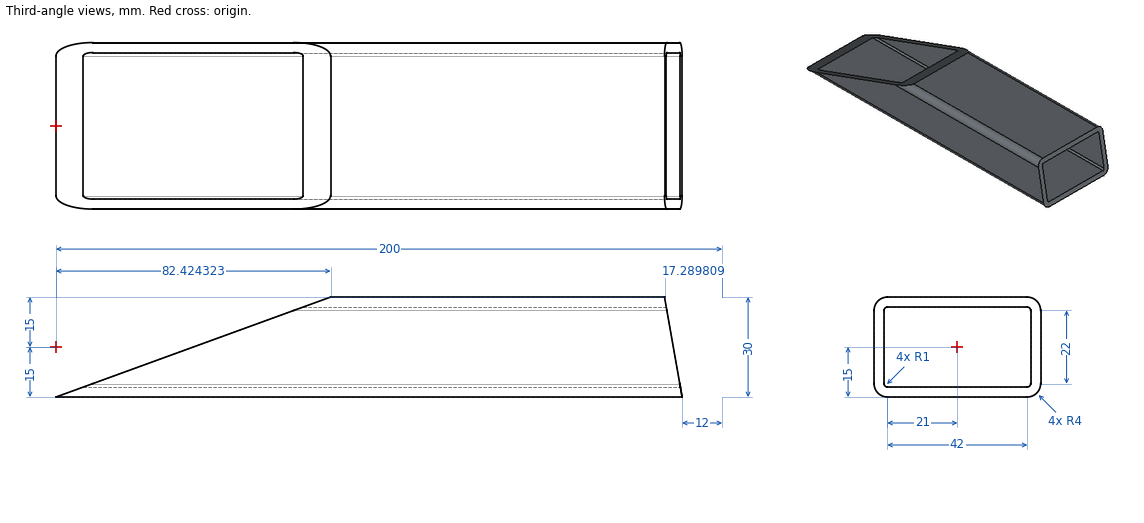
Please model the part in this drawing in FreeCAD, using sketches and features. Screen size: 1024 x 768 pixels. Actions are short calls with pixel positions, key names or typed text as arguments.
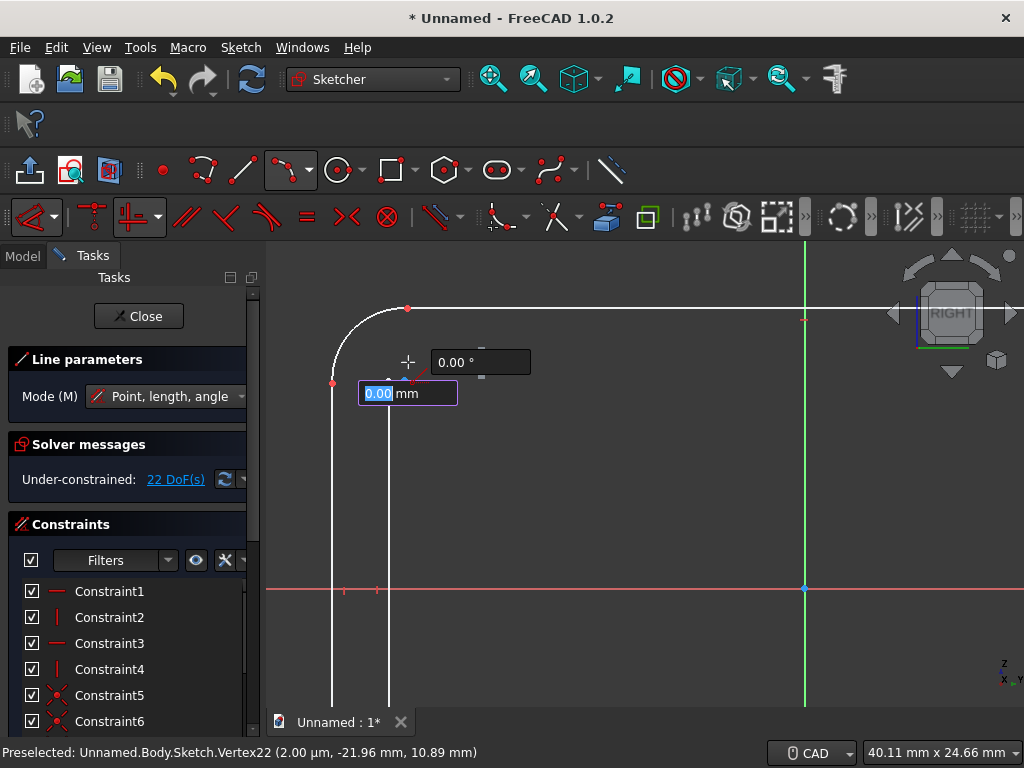
scroll(390, 380, down, 4)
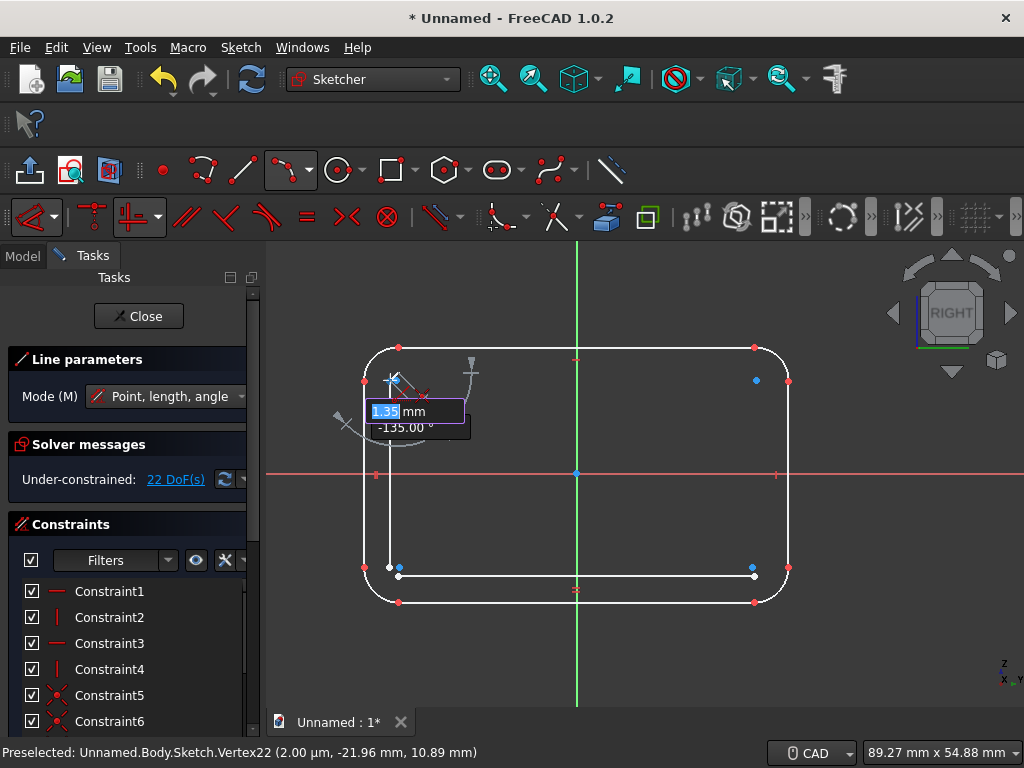
scroll(755, 372, up, 4)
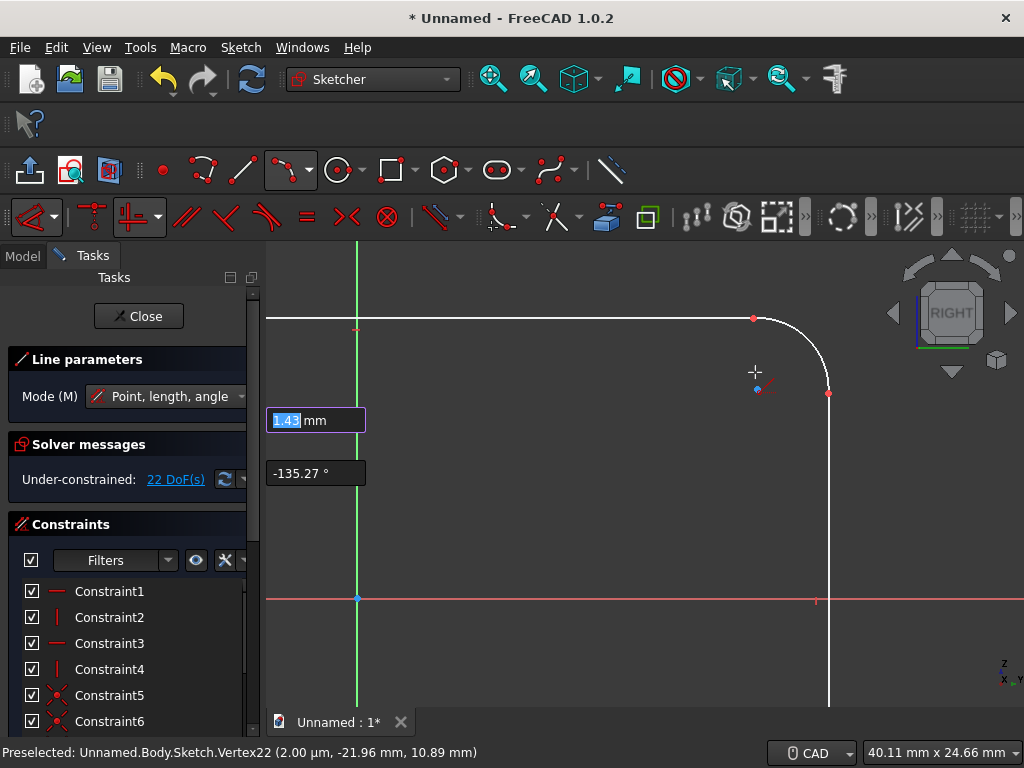
click(754, 372)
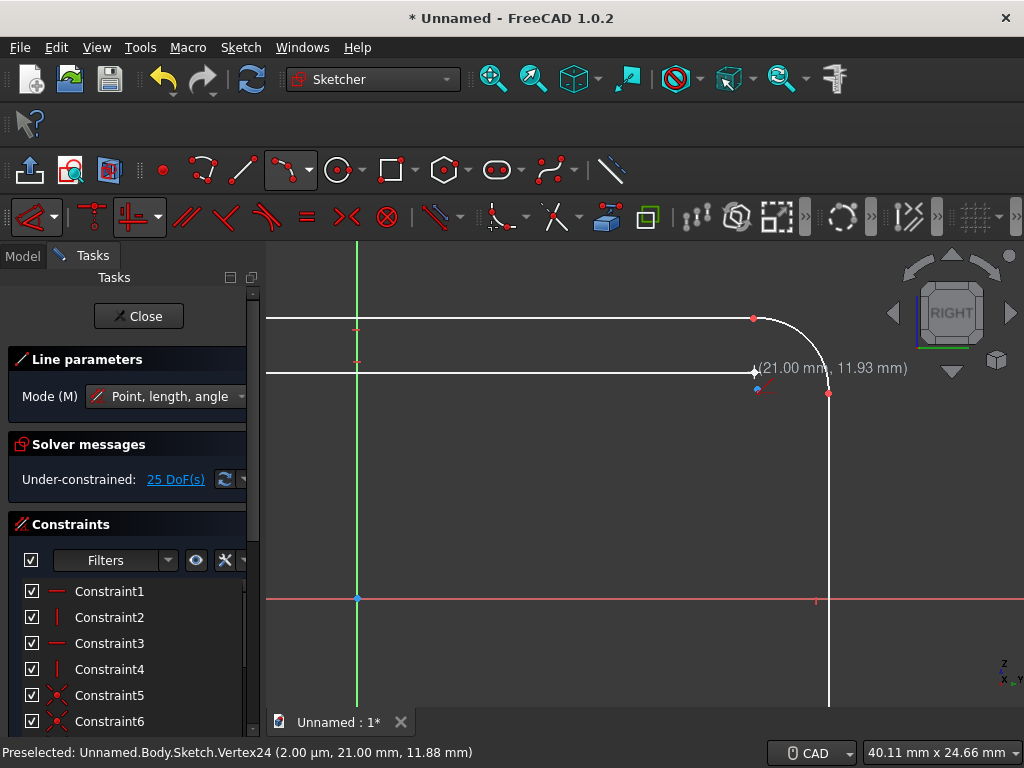
click(773, 391)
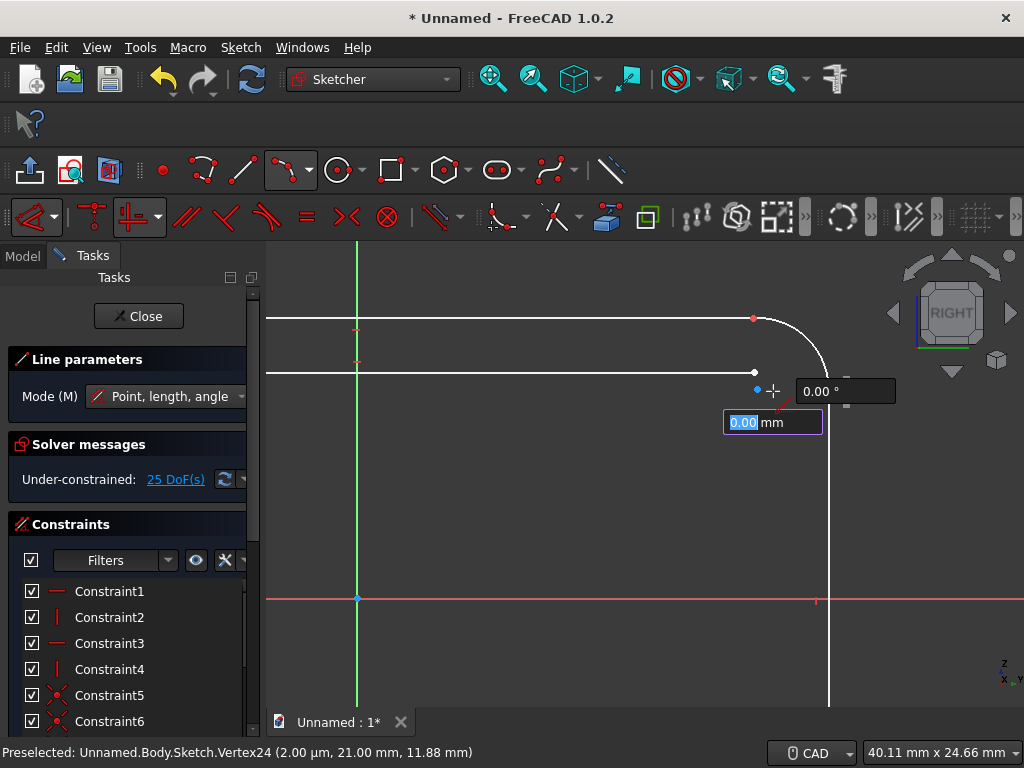
scroll(756, 372, down, 4)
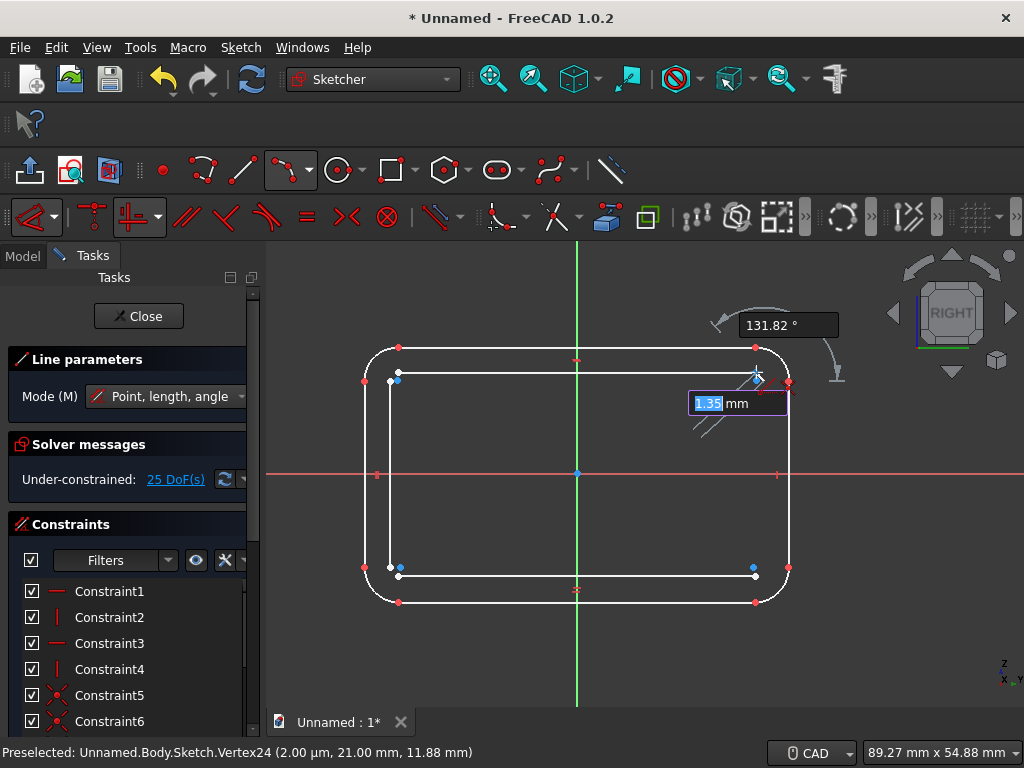
scroll(764, 567, up, 4)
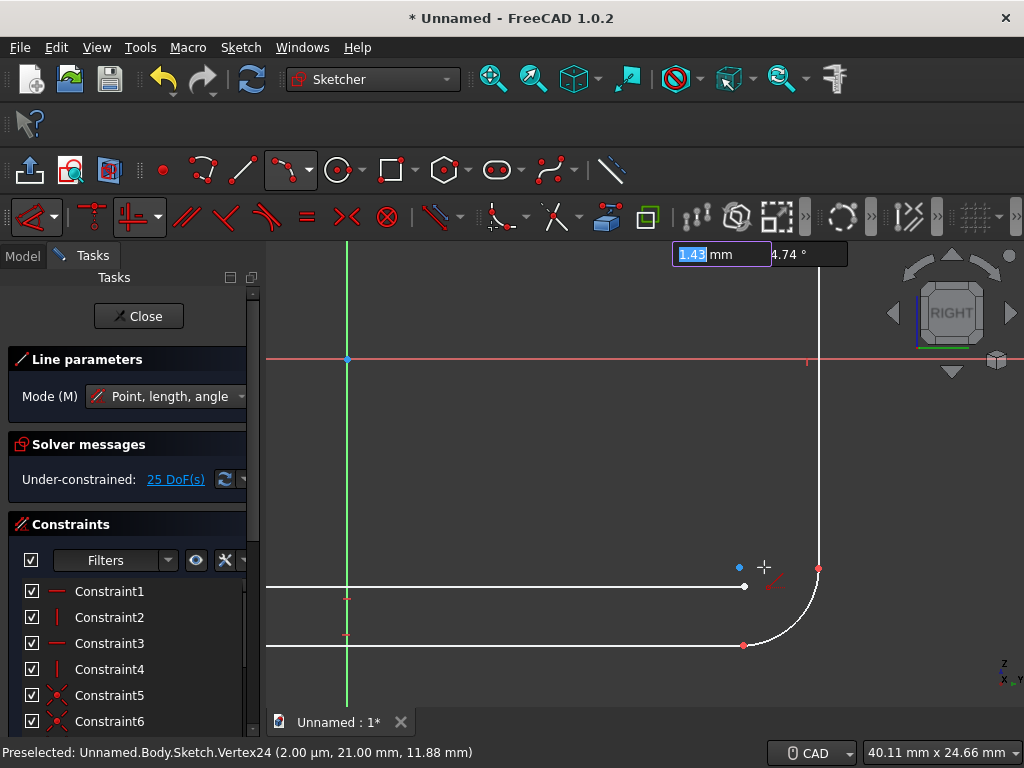
click(763, 567)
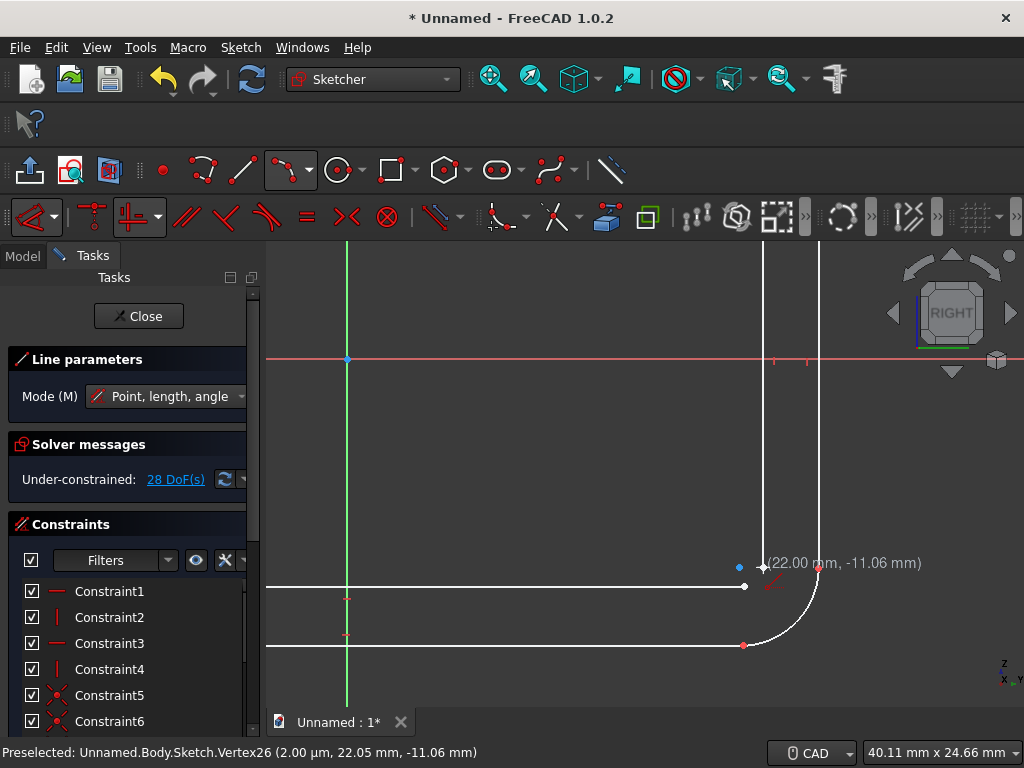
click(284, 170)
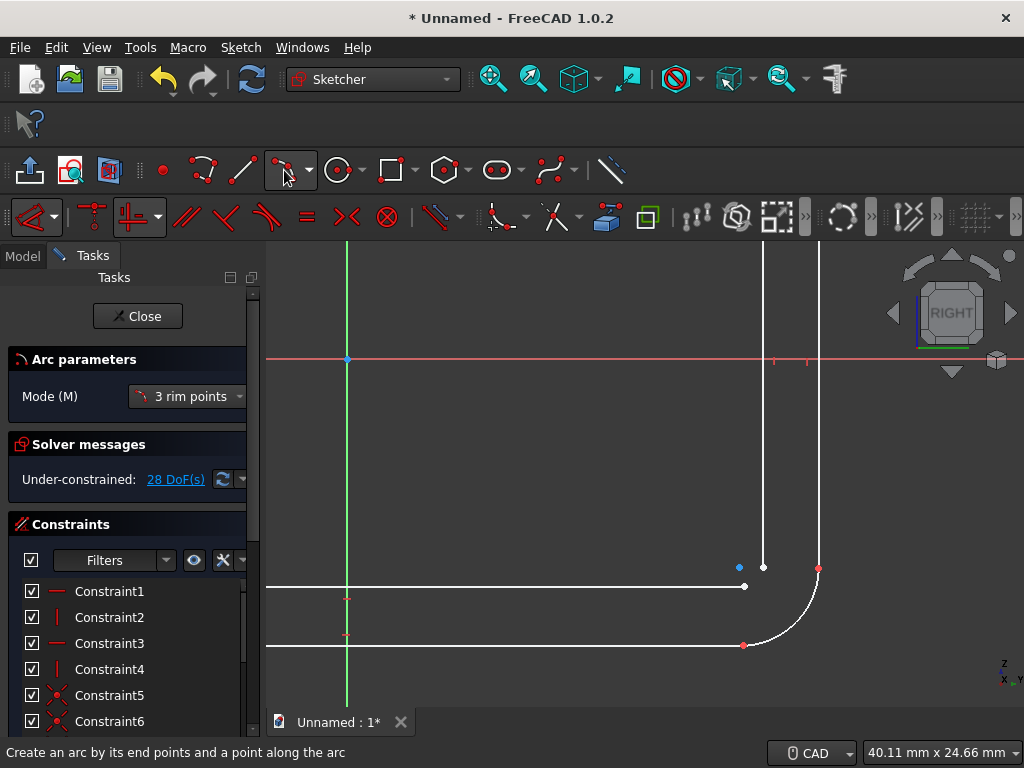
scroll(764, 568, down, 4)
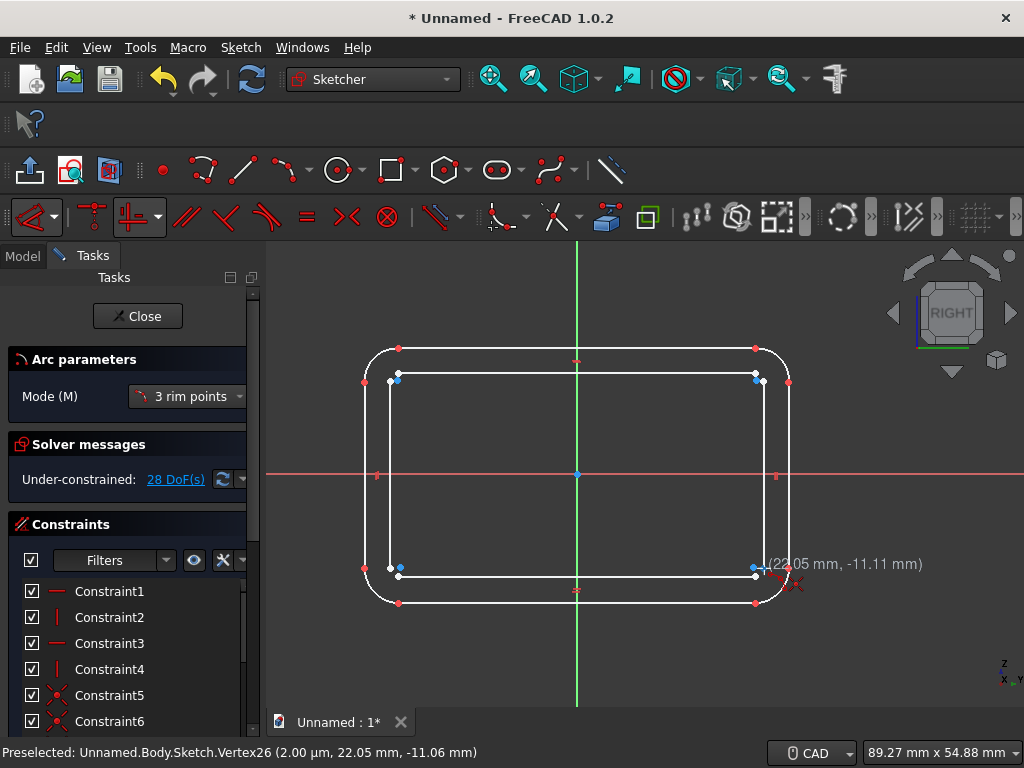
scroll(399, 576, up, 4)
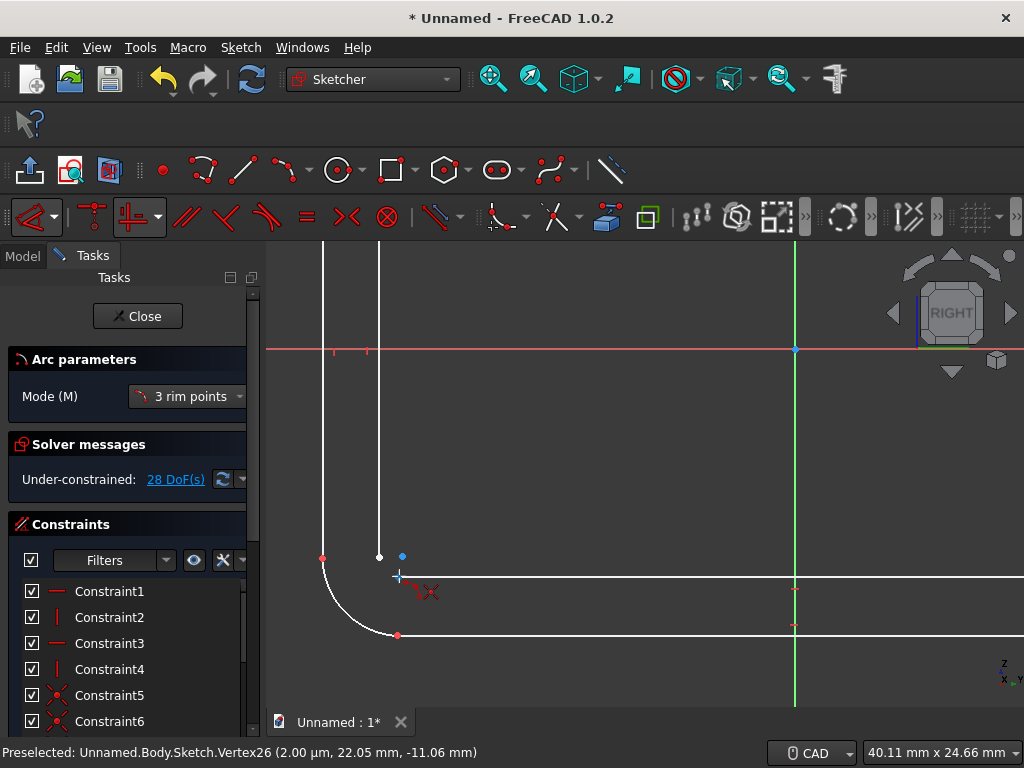
click(398, 577)
click(379, 558)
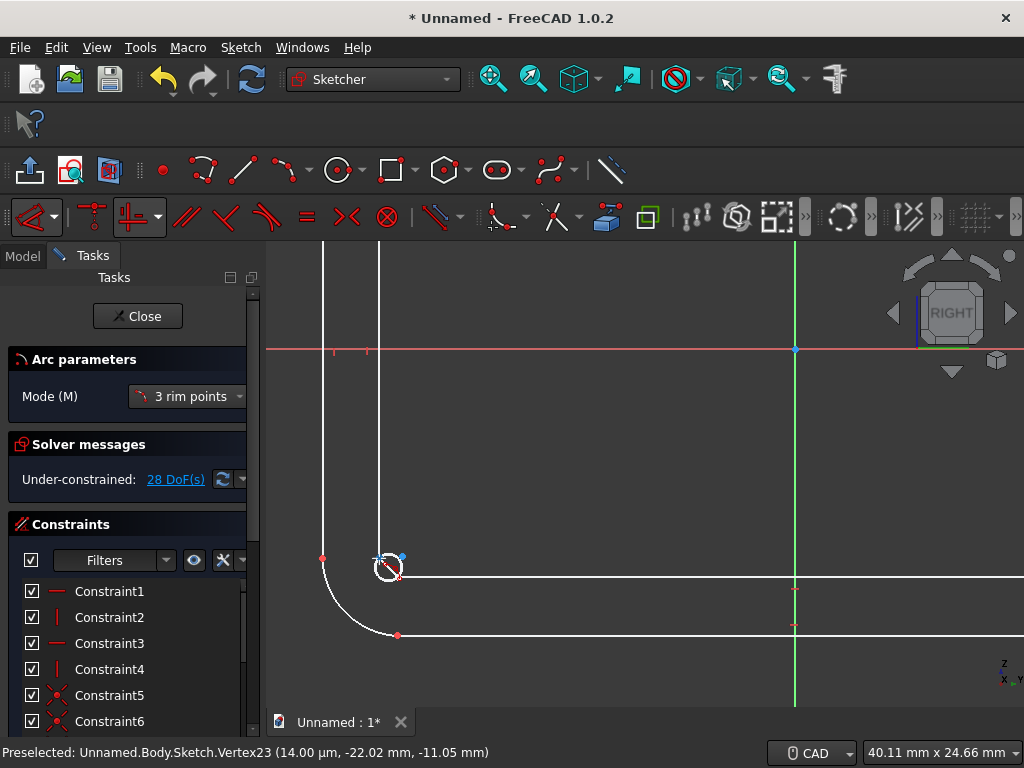
scroll(385, 570, up, 6)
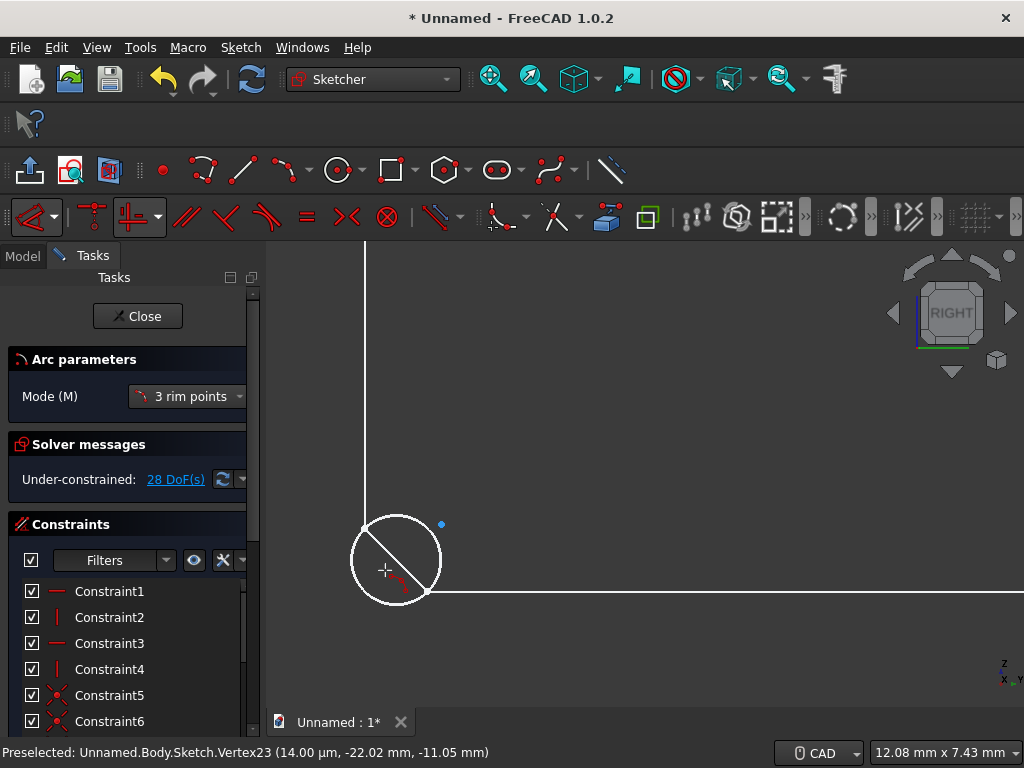
click(385, 570)